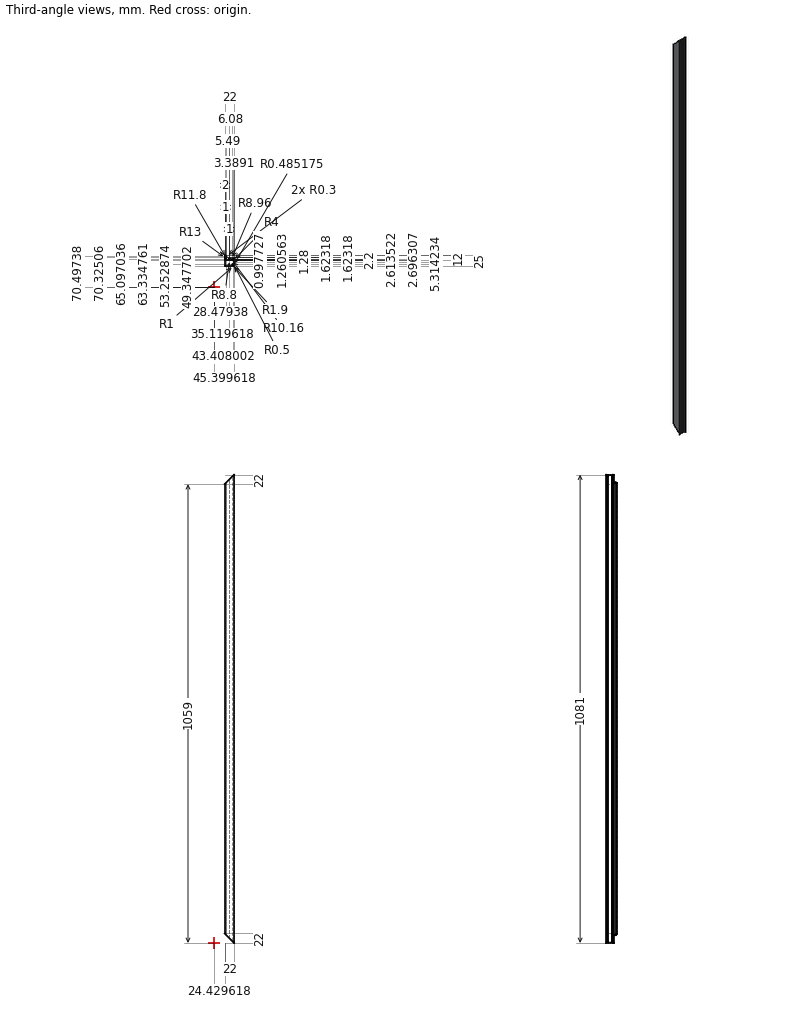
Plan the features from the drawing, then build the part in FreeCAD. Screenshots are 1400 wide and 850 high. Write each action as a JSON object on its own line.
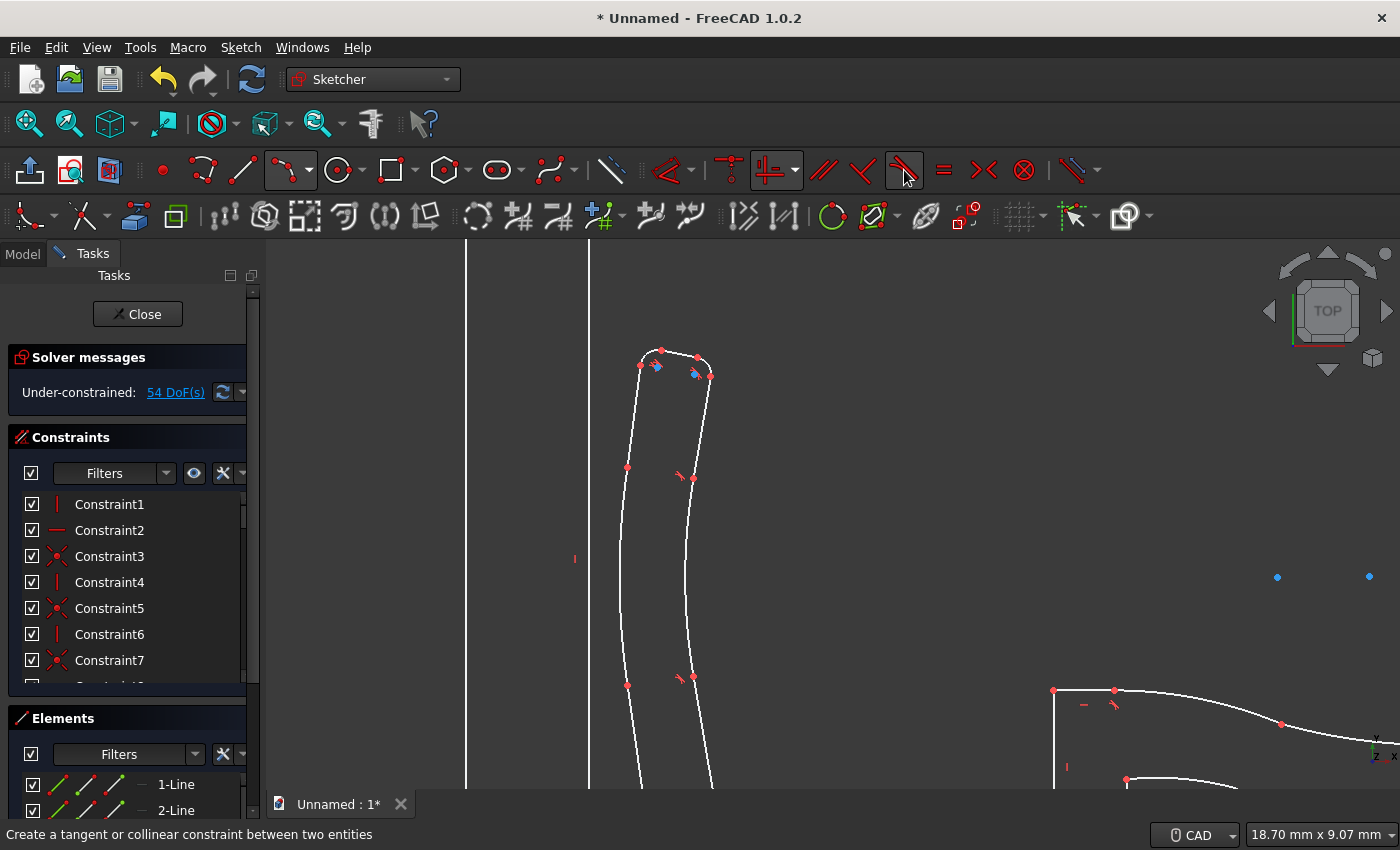
{"action": "left_click", "coordinate": [637, 396]}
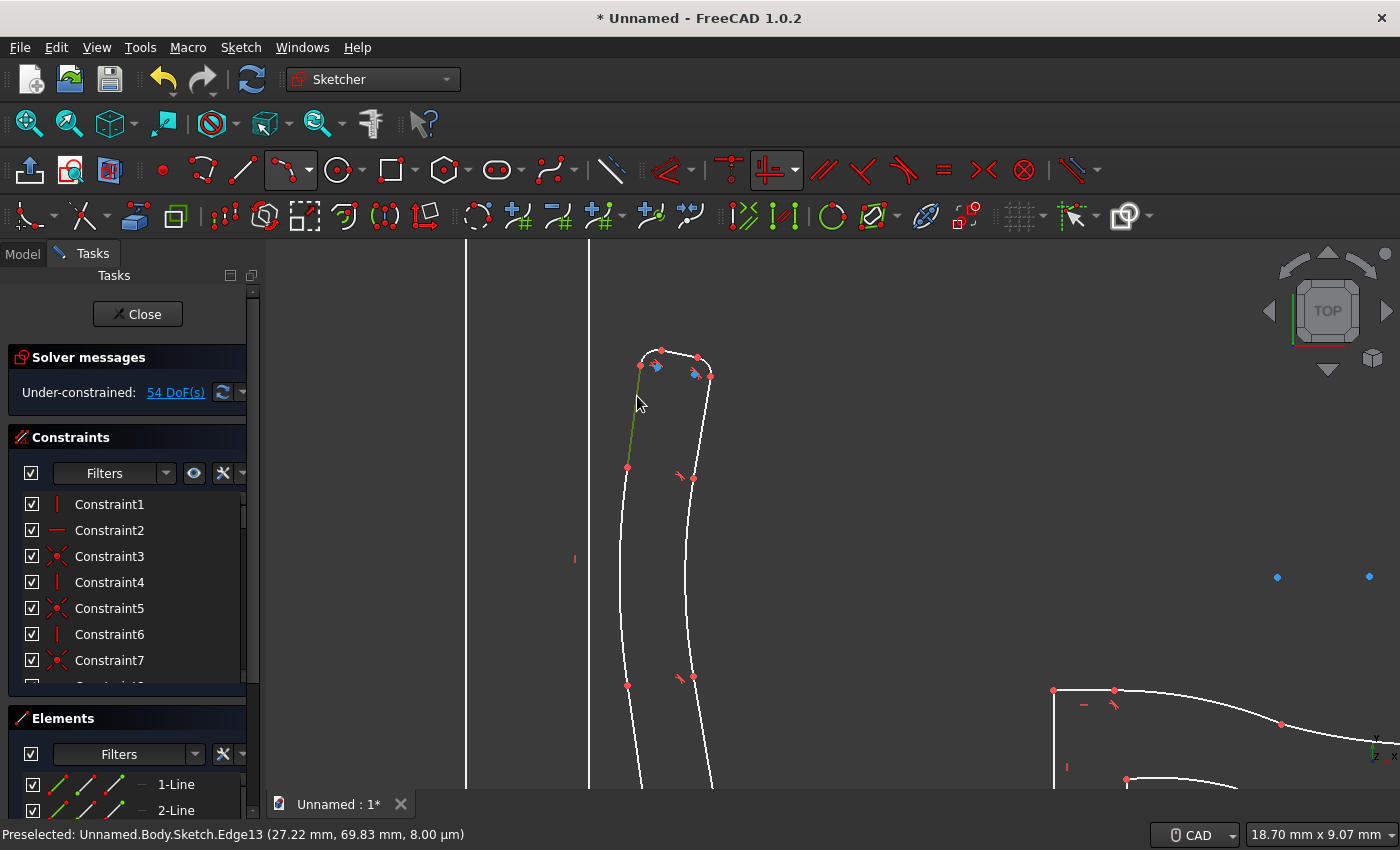
{"action": "left_click", "coordinate": [621, 533]}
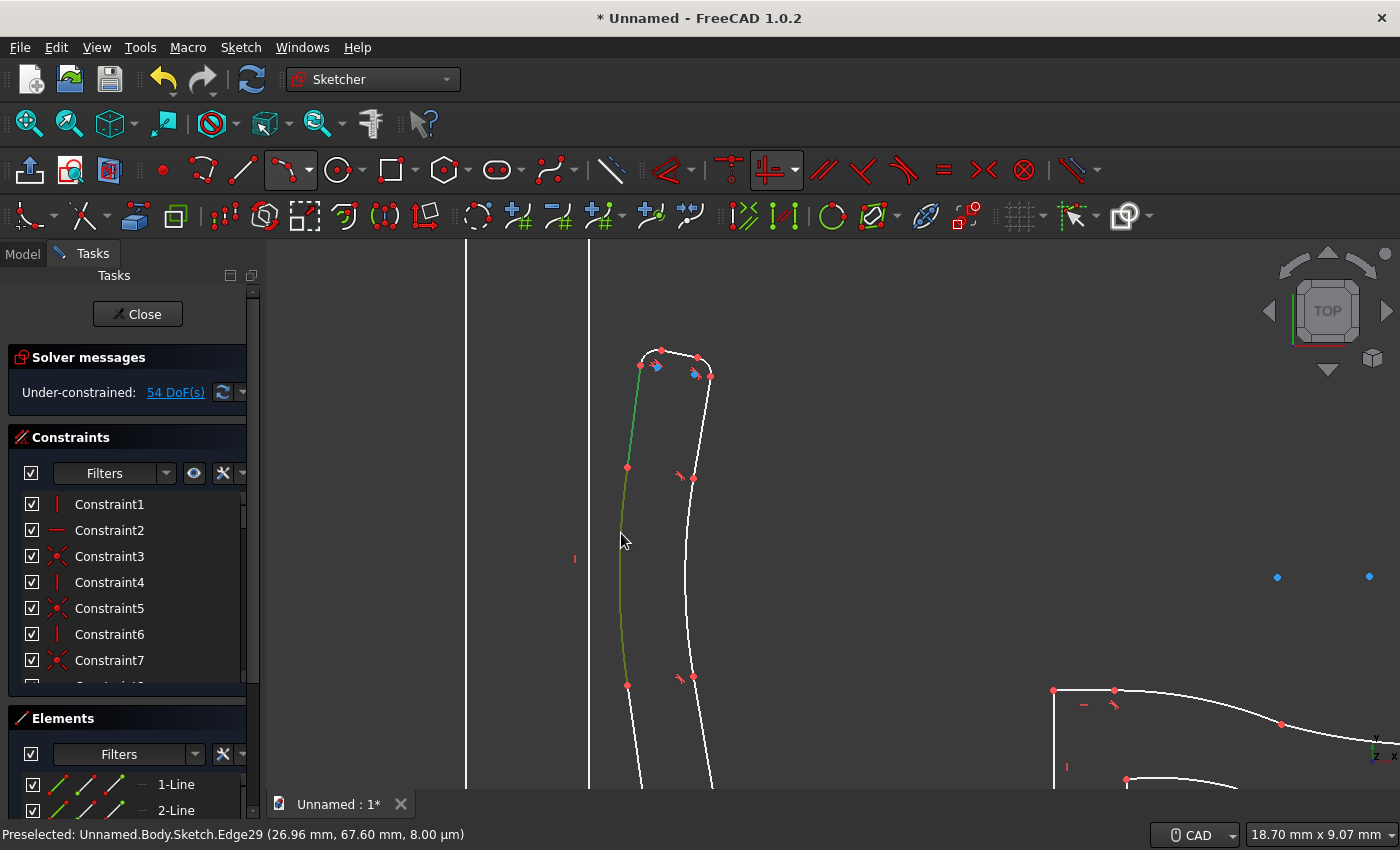
{"action": "left_click", "coordinate": [904, 170]}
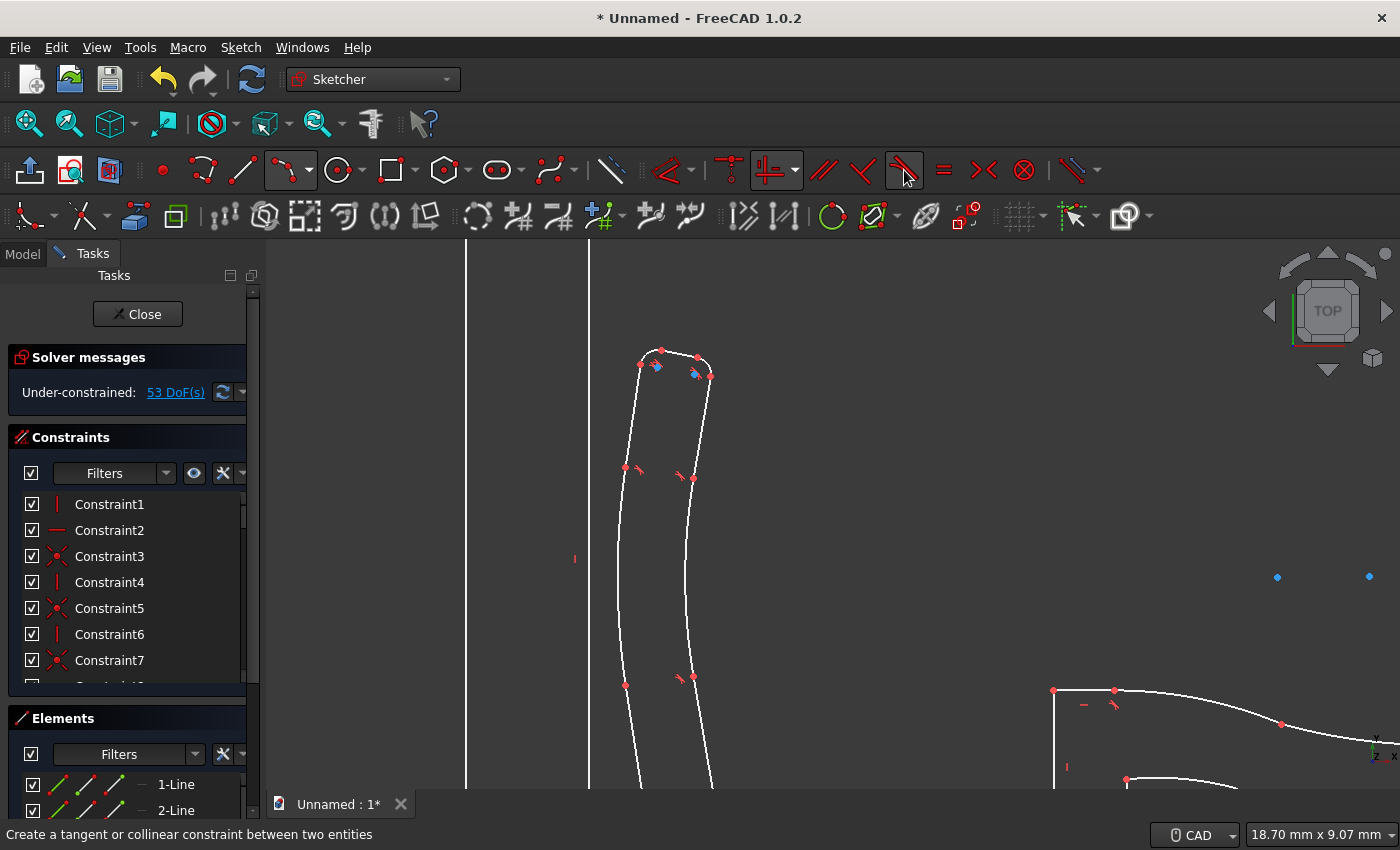
{"action": "scroll", "coordinate": [643, 371], "scroll_direction": "down", "scroll_amount": 7}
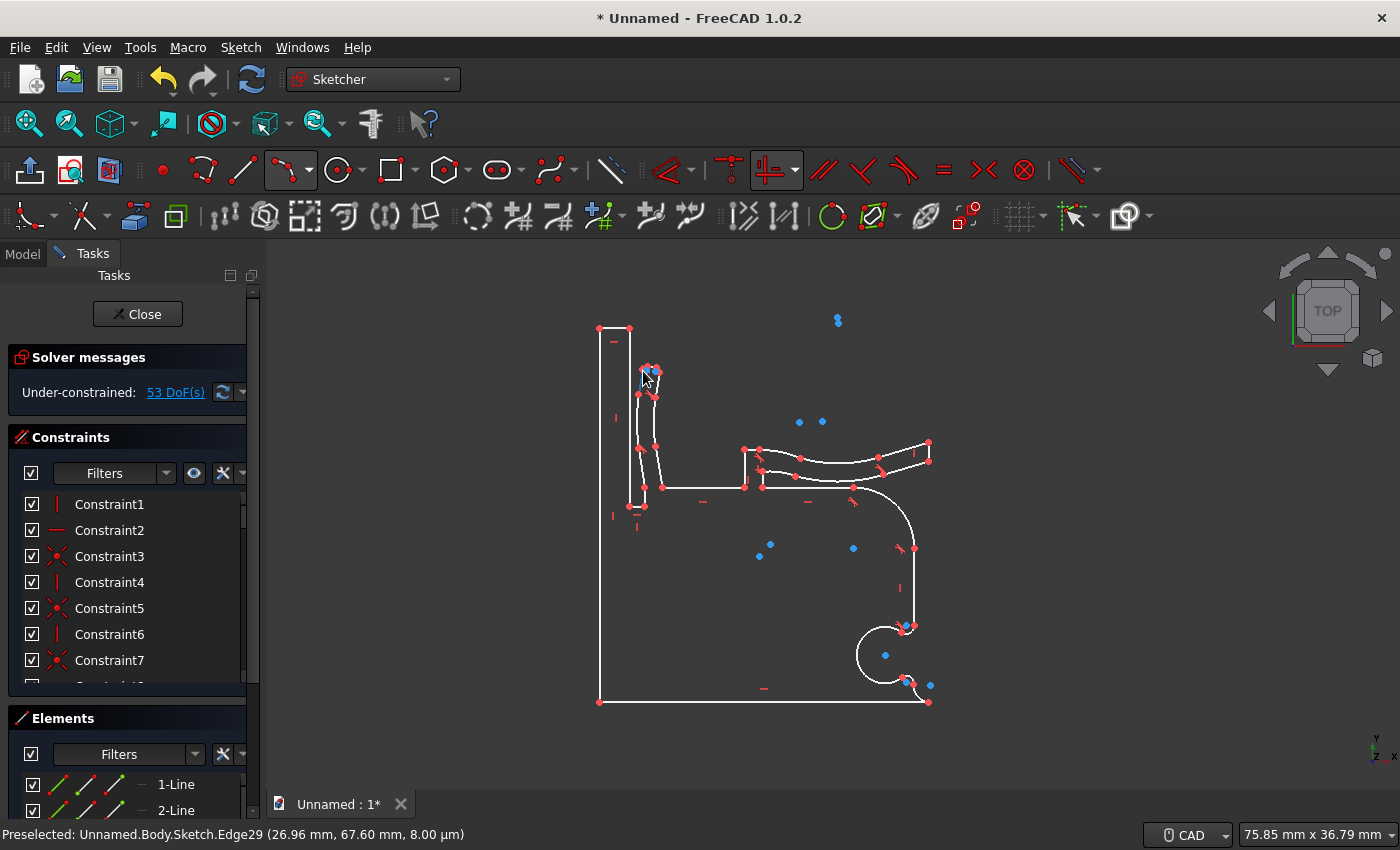
{"action": "scroll", "coordinate": [641, 460], "scroll_direction": "up", "scroll_amount": 2}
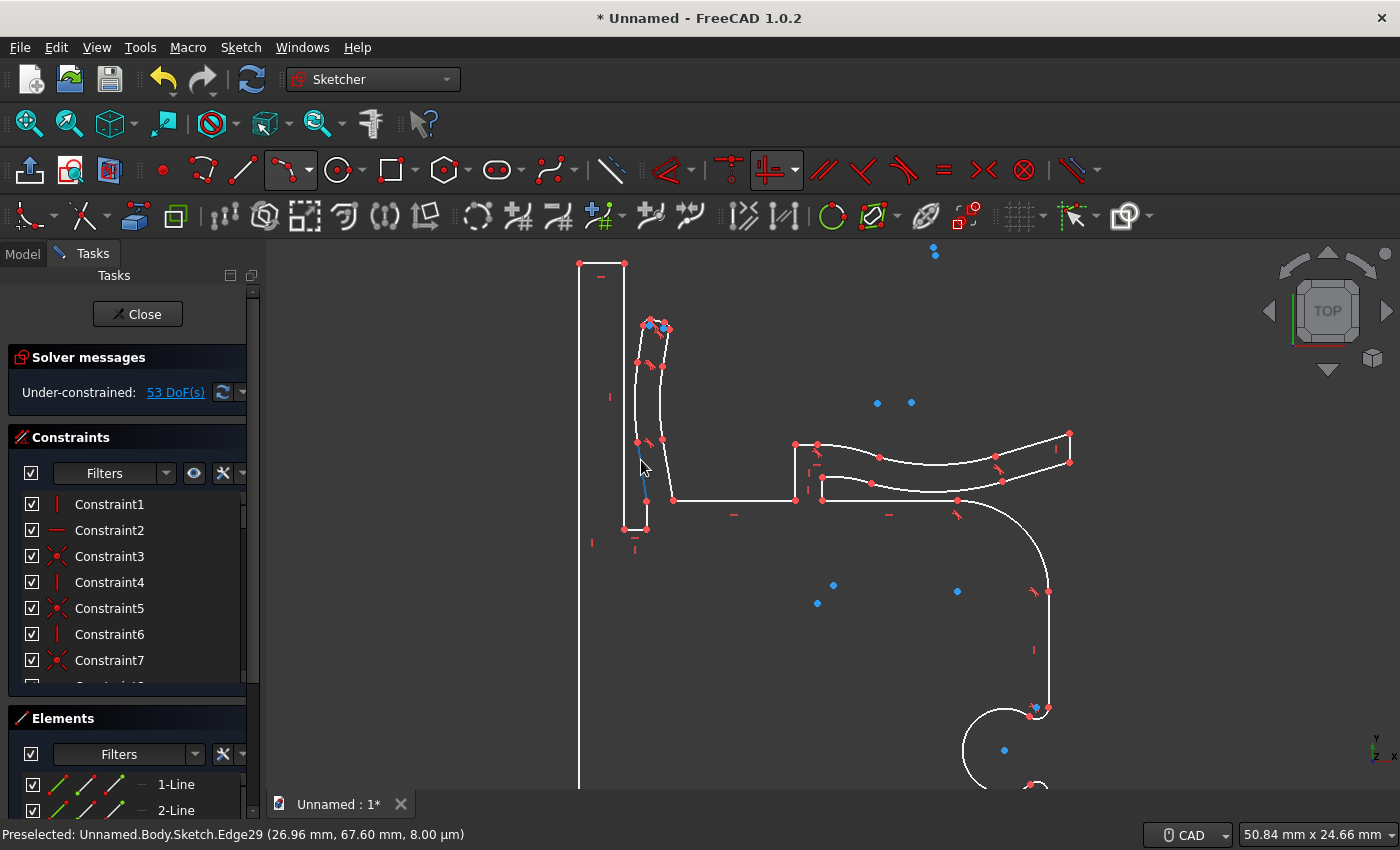
{"action": "left_click", "coordinate": [640, 460]}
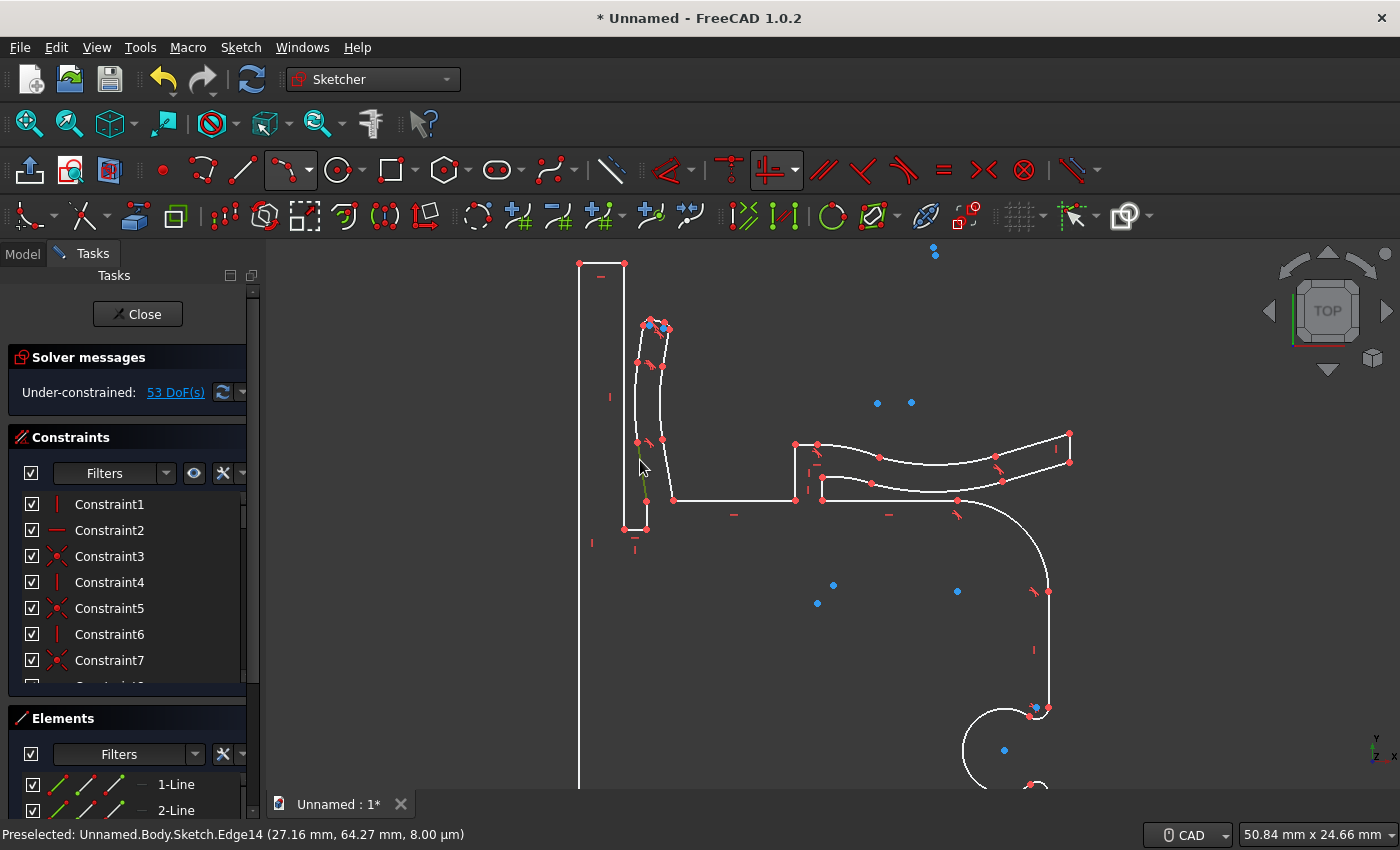
{"action": "scroll", "coordinate": [635, 387], "scroll_direction": "up", "scroll_amount": 2}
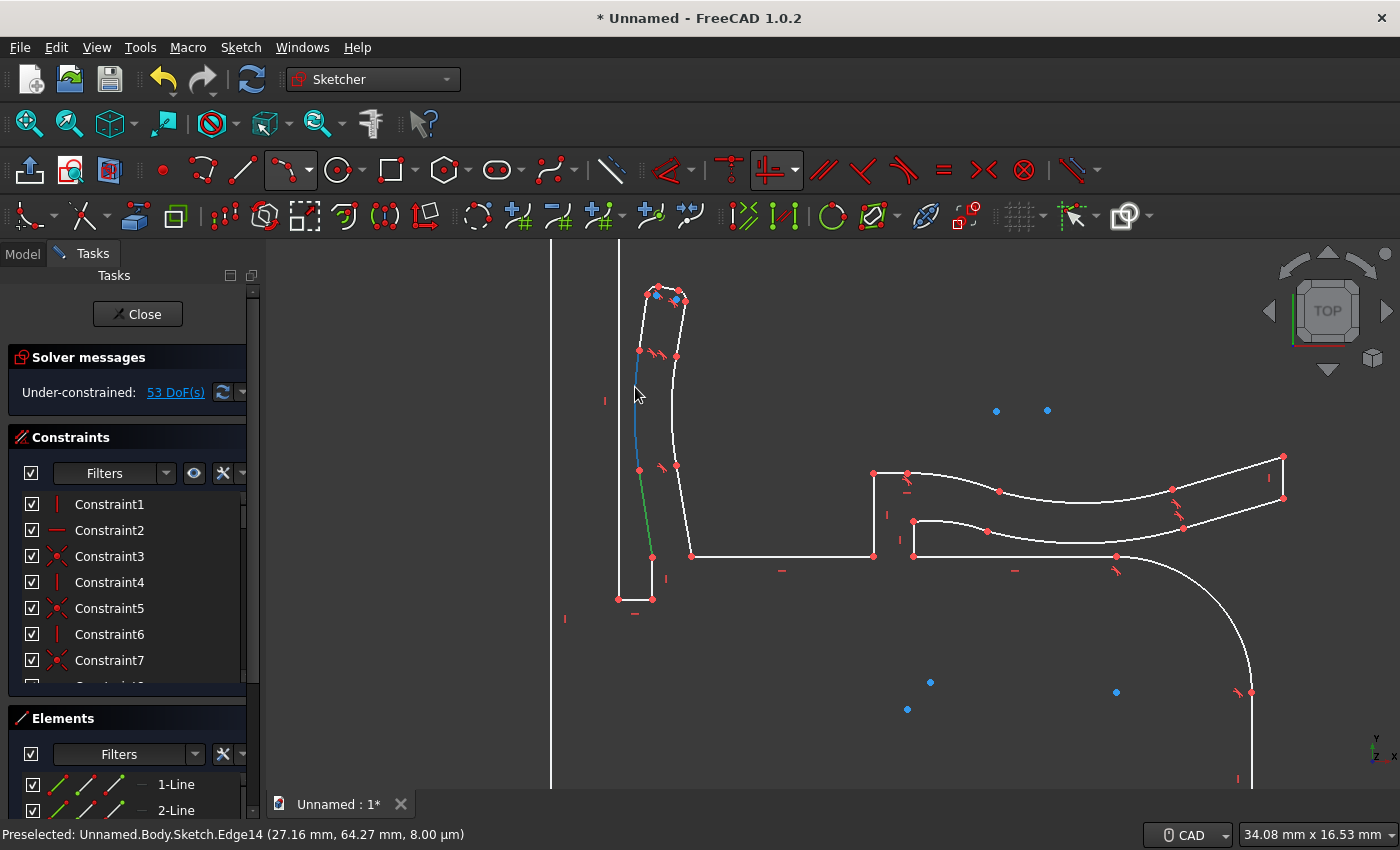
{"action": "left_click", "coordinate": [635, 386]}